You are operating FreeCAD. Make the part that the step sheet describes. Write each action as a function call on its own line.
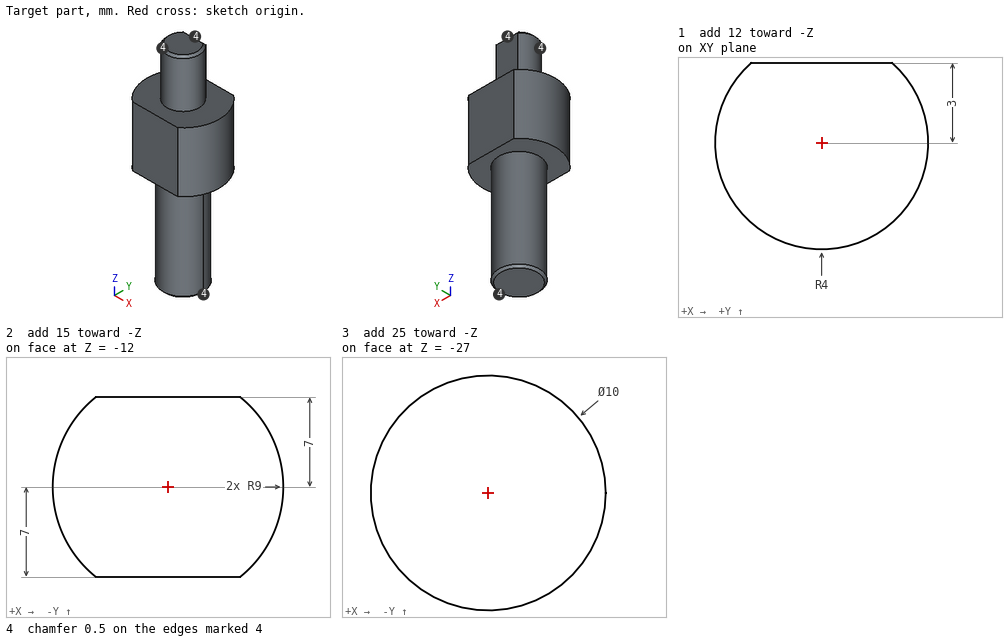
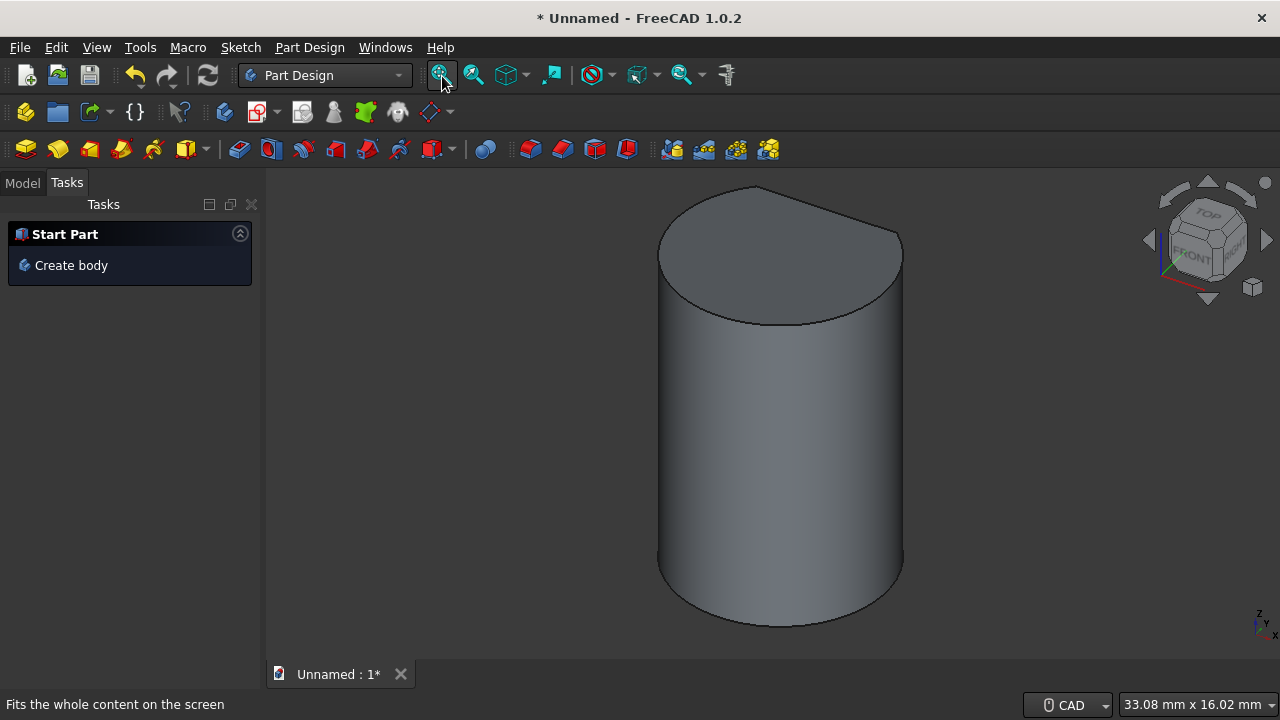
key(5)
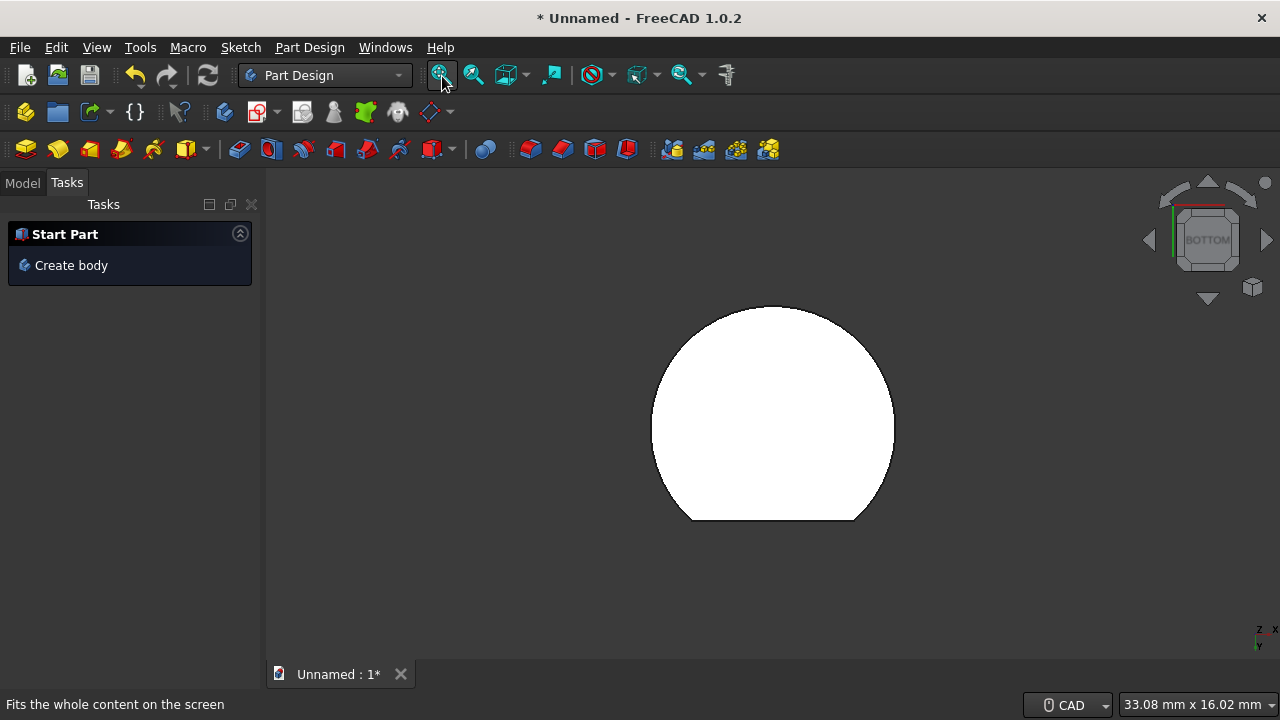
key(v)
key(f)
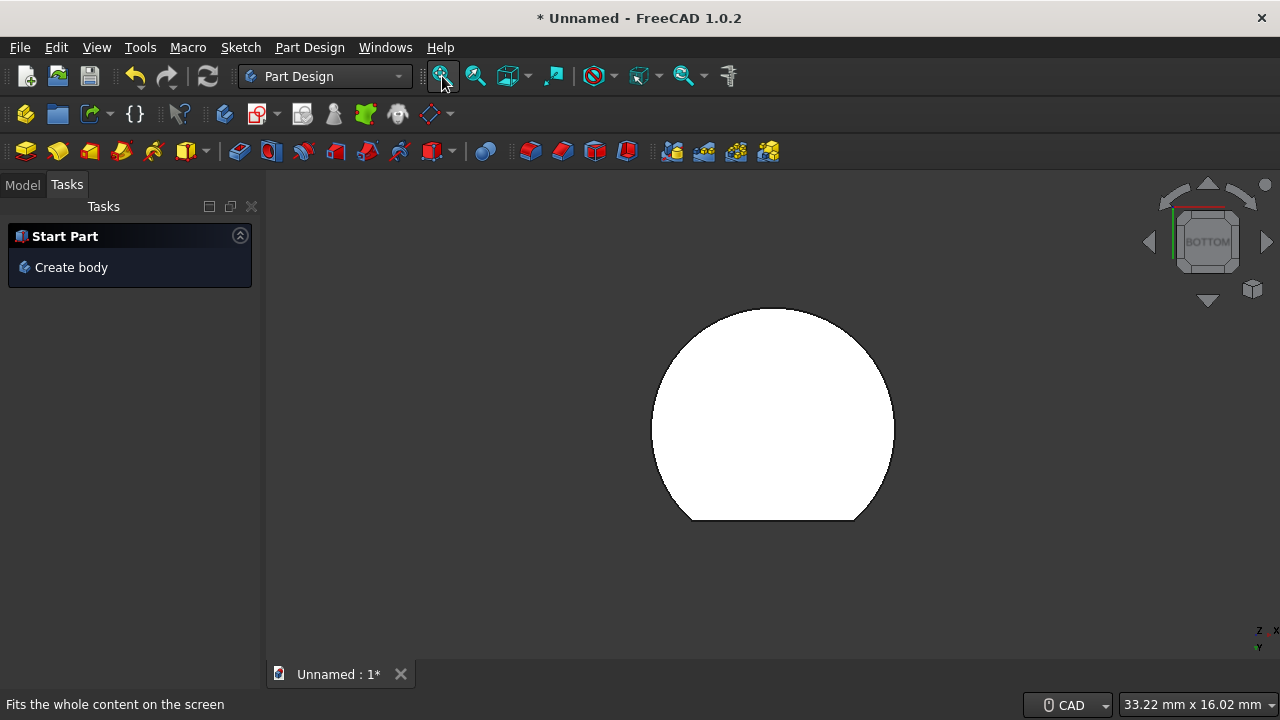
click(773, 413)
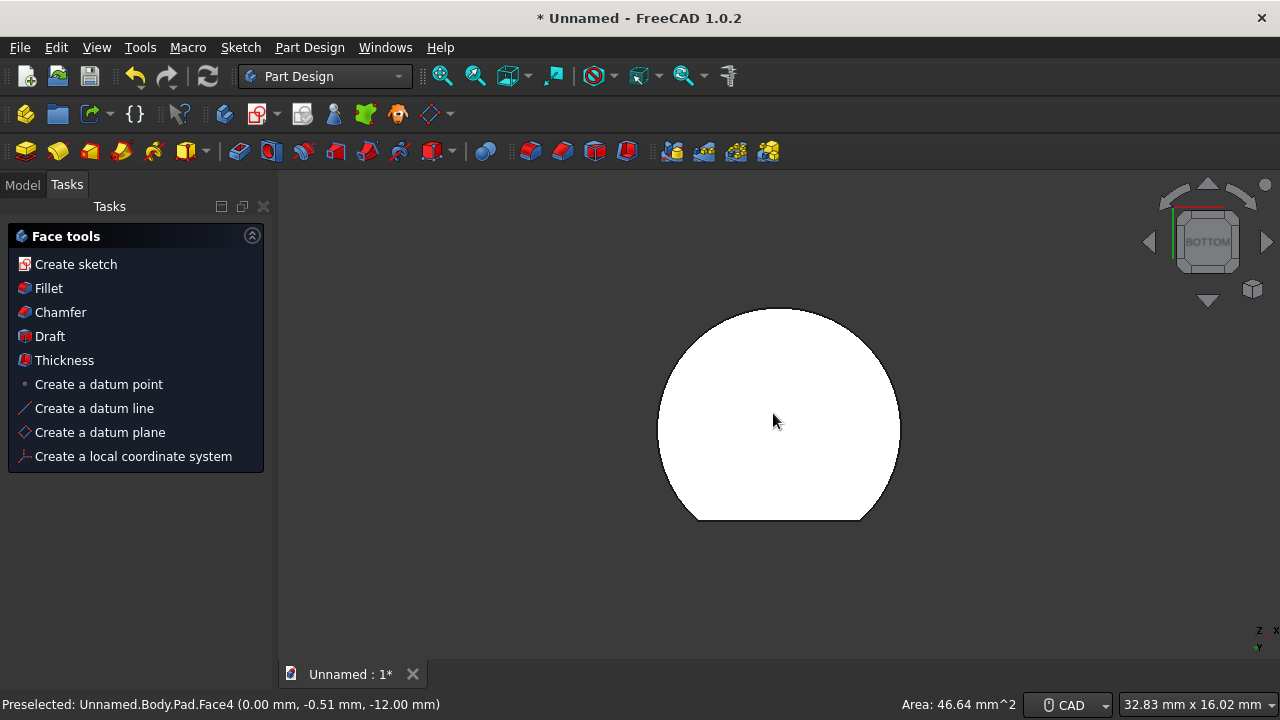
click(258, 114)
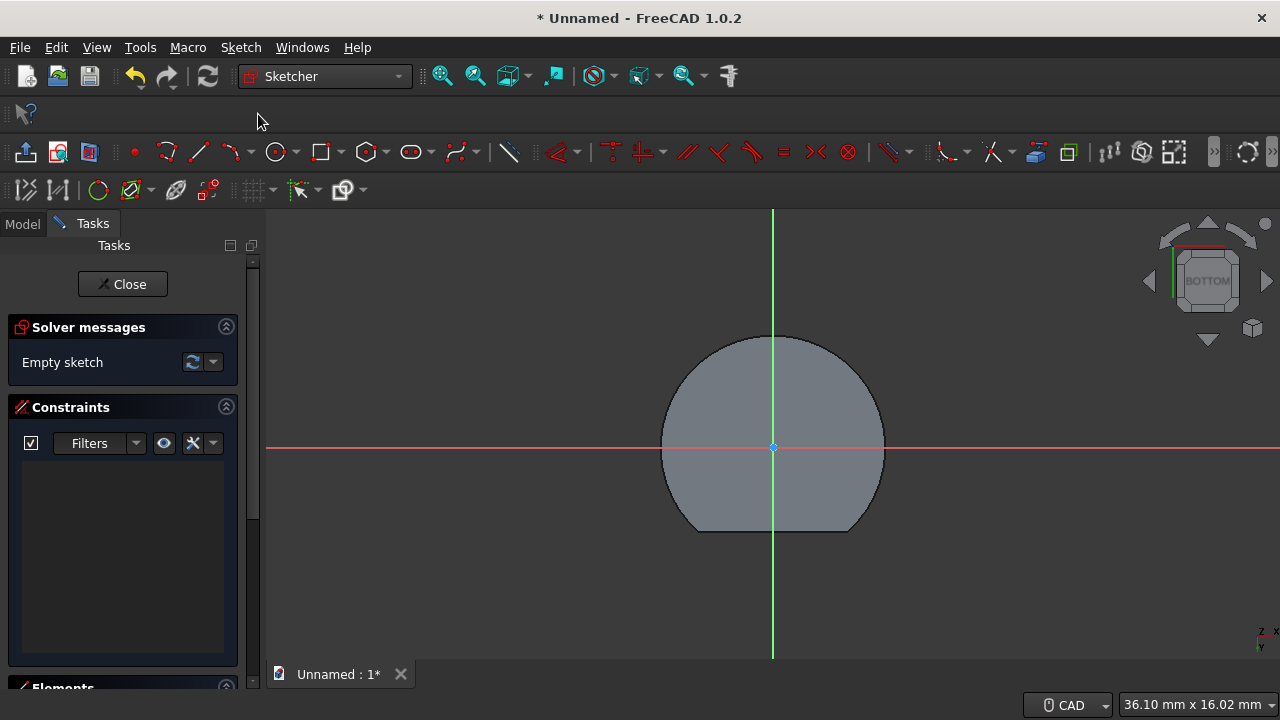
scroll(565, 406, down, 2)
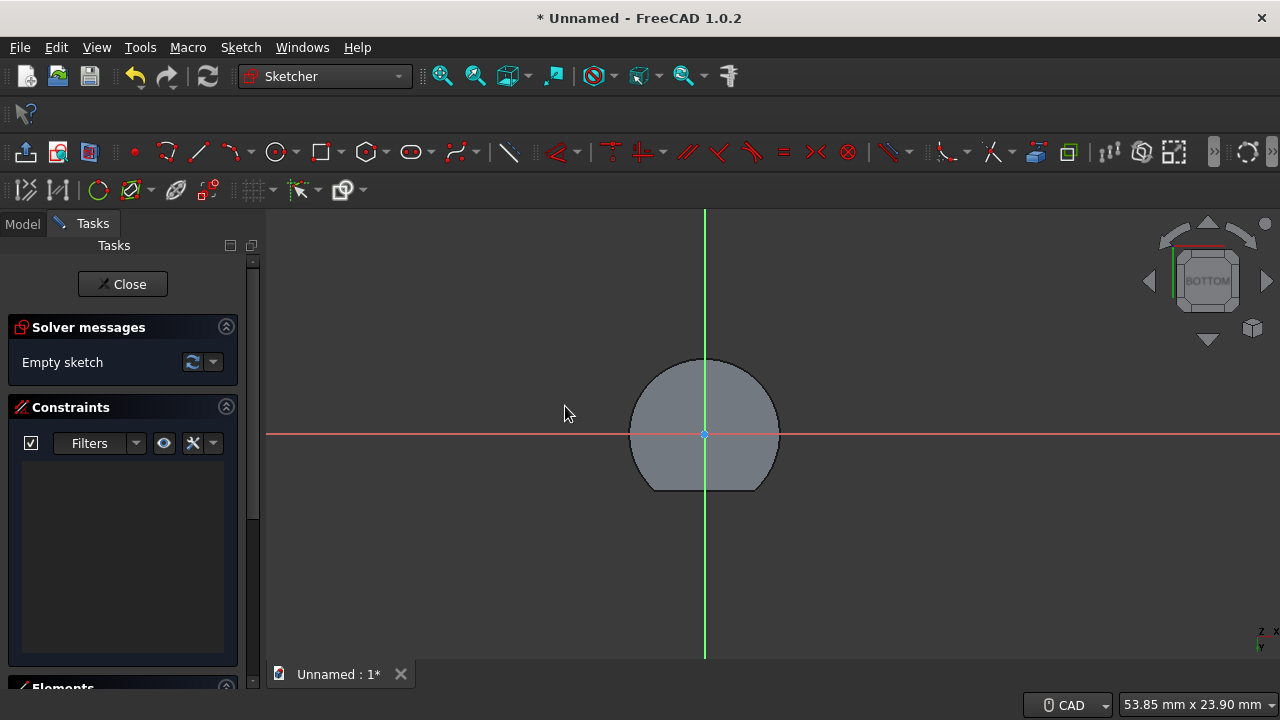
key(g)
key(l)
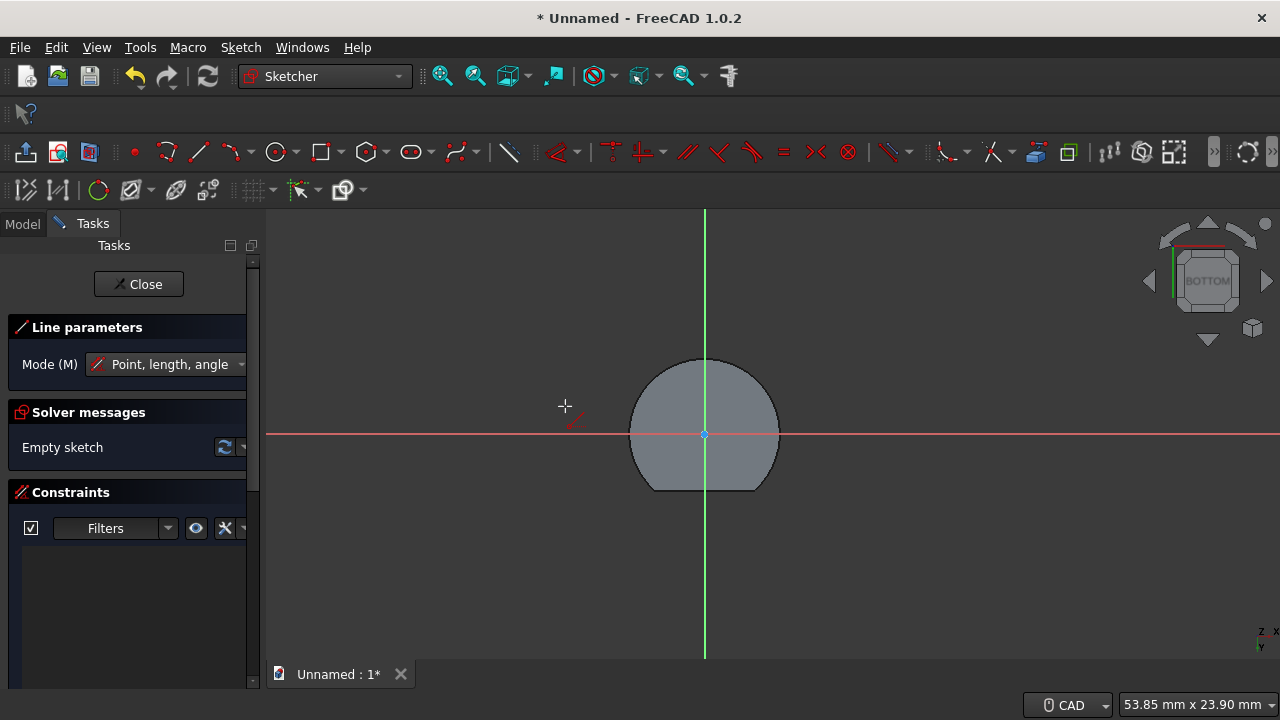
click(598, 566)
click(811, 566)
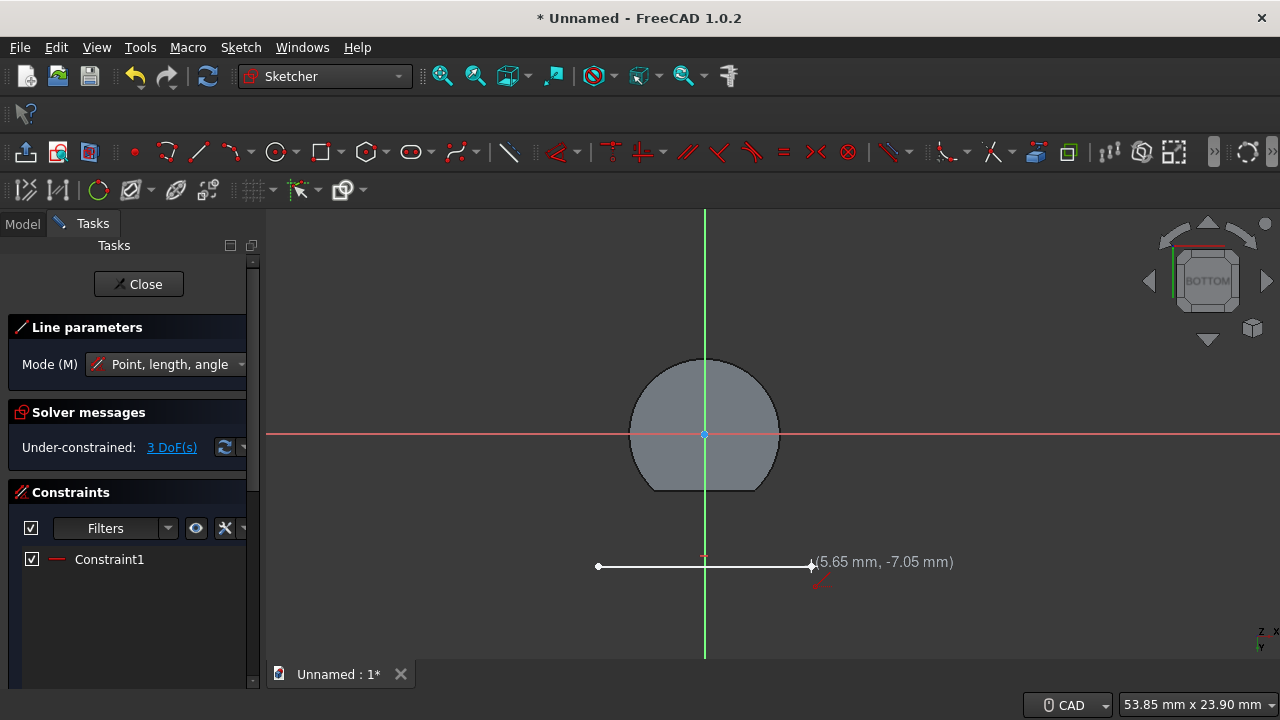
click(811, 302)
click(598, 302)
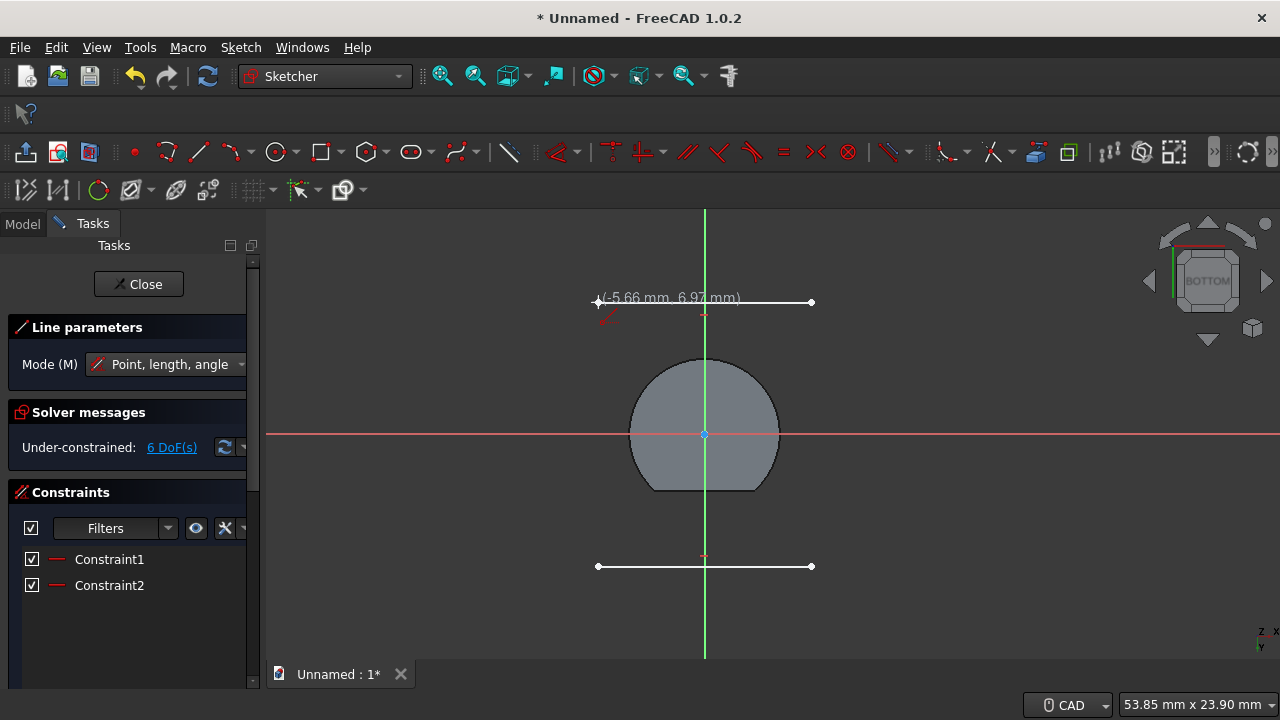
key(g)
key(3)
key(a)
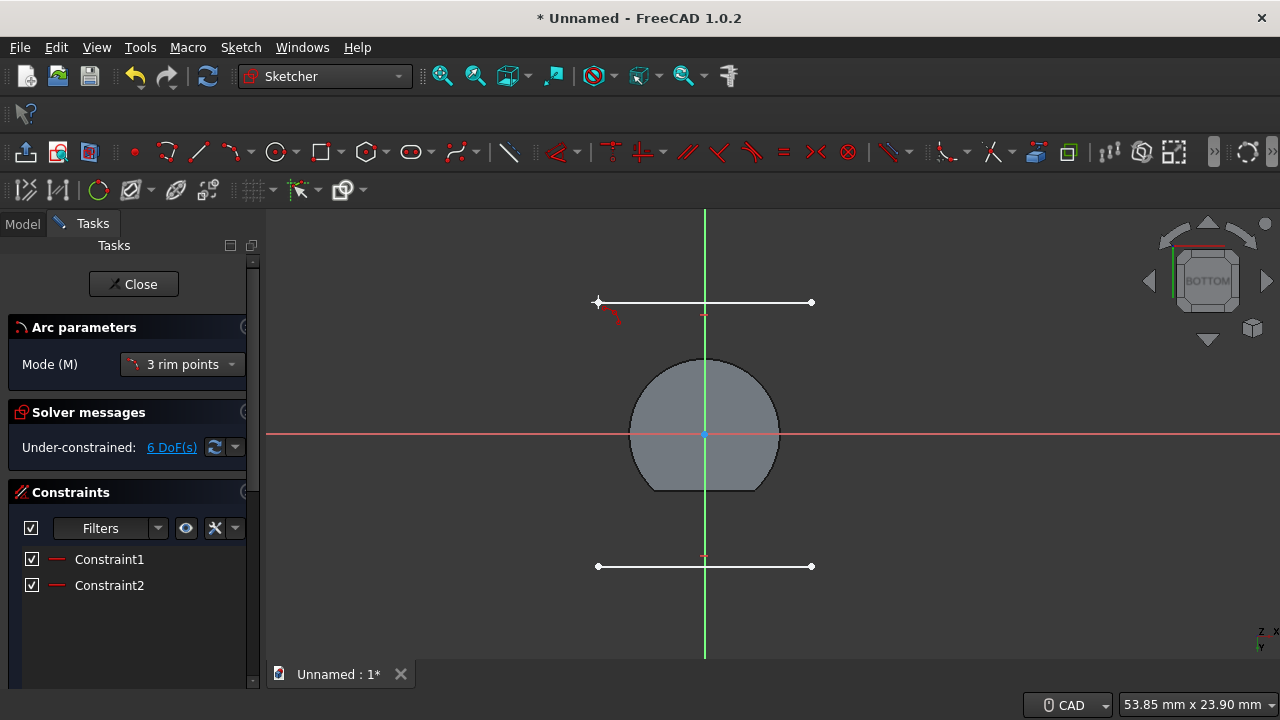
click(811, 567)
click(811, 303)
click(871, 464)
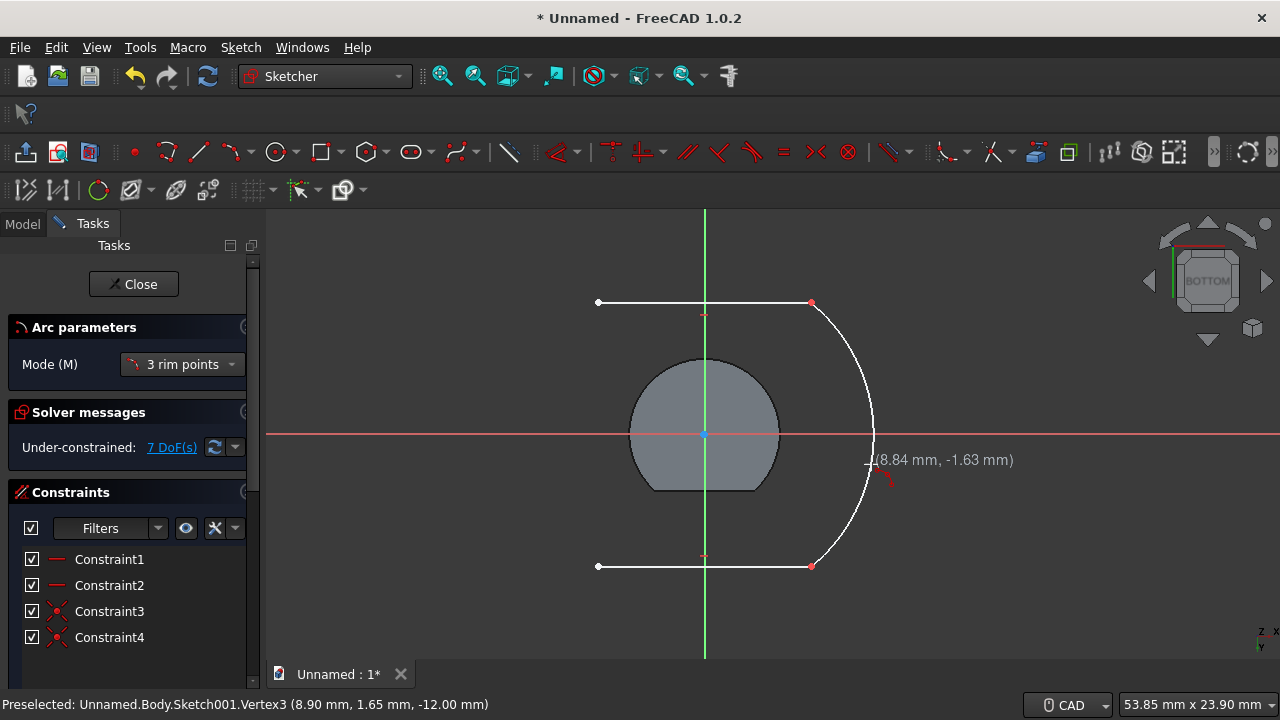
click(598, 303)
click(598, 567)
click(538, 404)
key(Escape)